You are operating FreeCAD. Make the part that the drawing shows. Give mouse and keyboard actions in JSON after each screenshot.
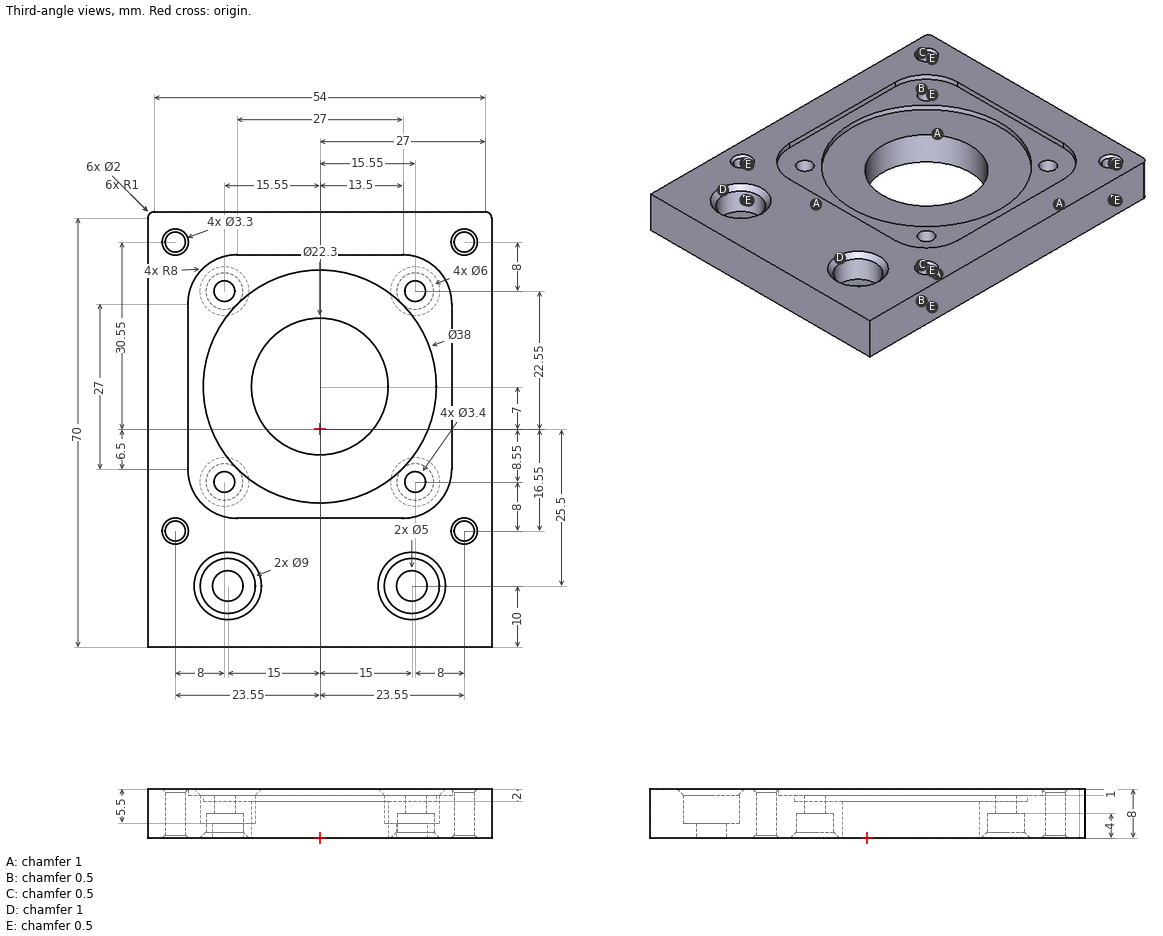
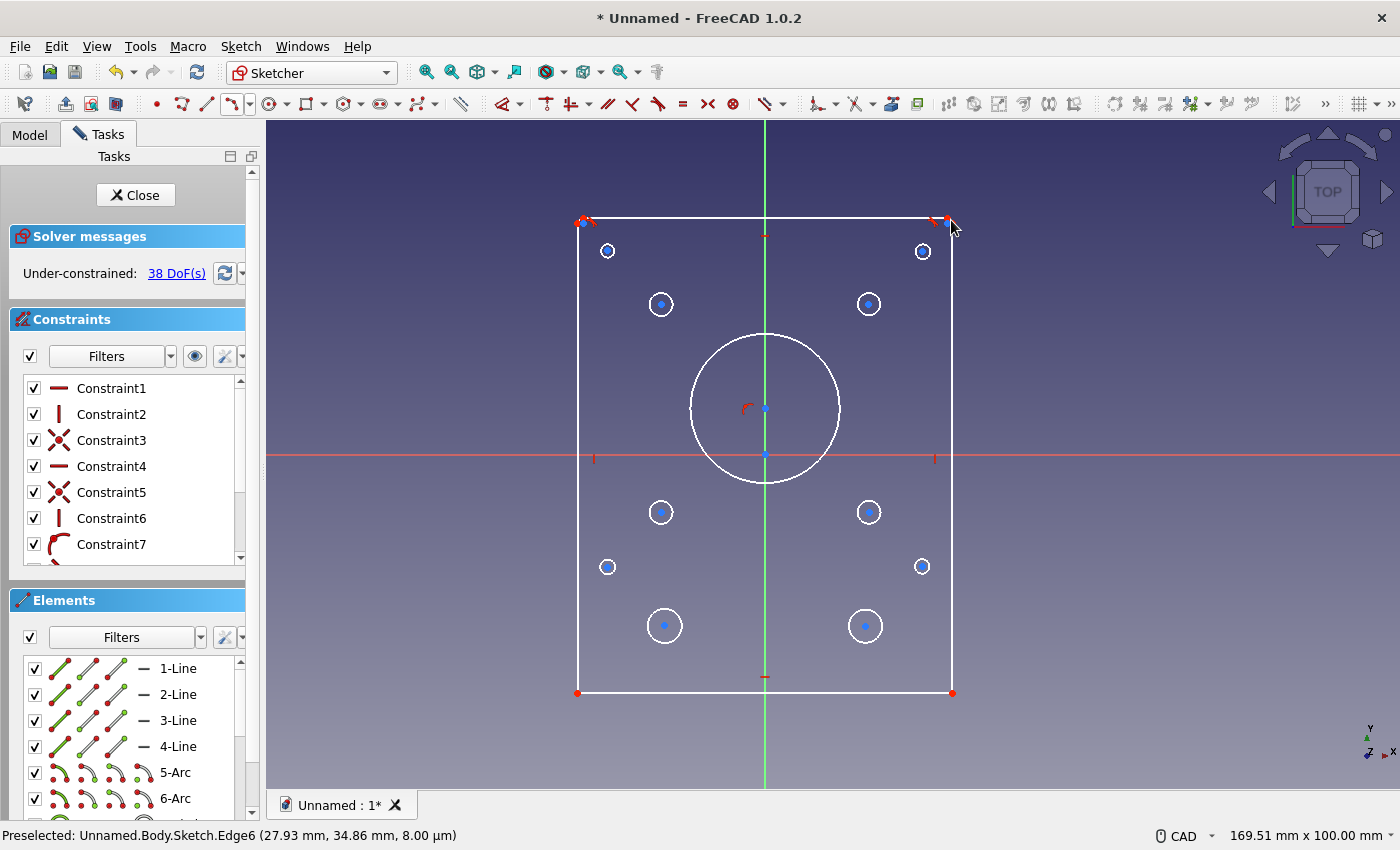
{"action": "scroll", "coordinate": [579, 220], "scroll_direction": "up", "scroll_amount": 7}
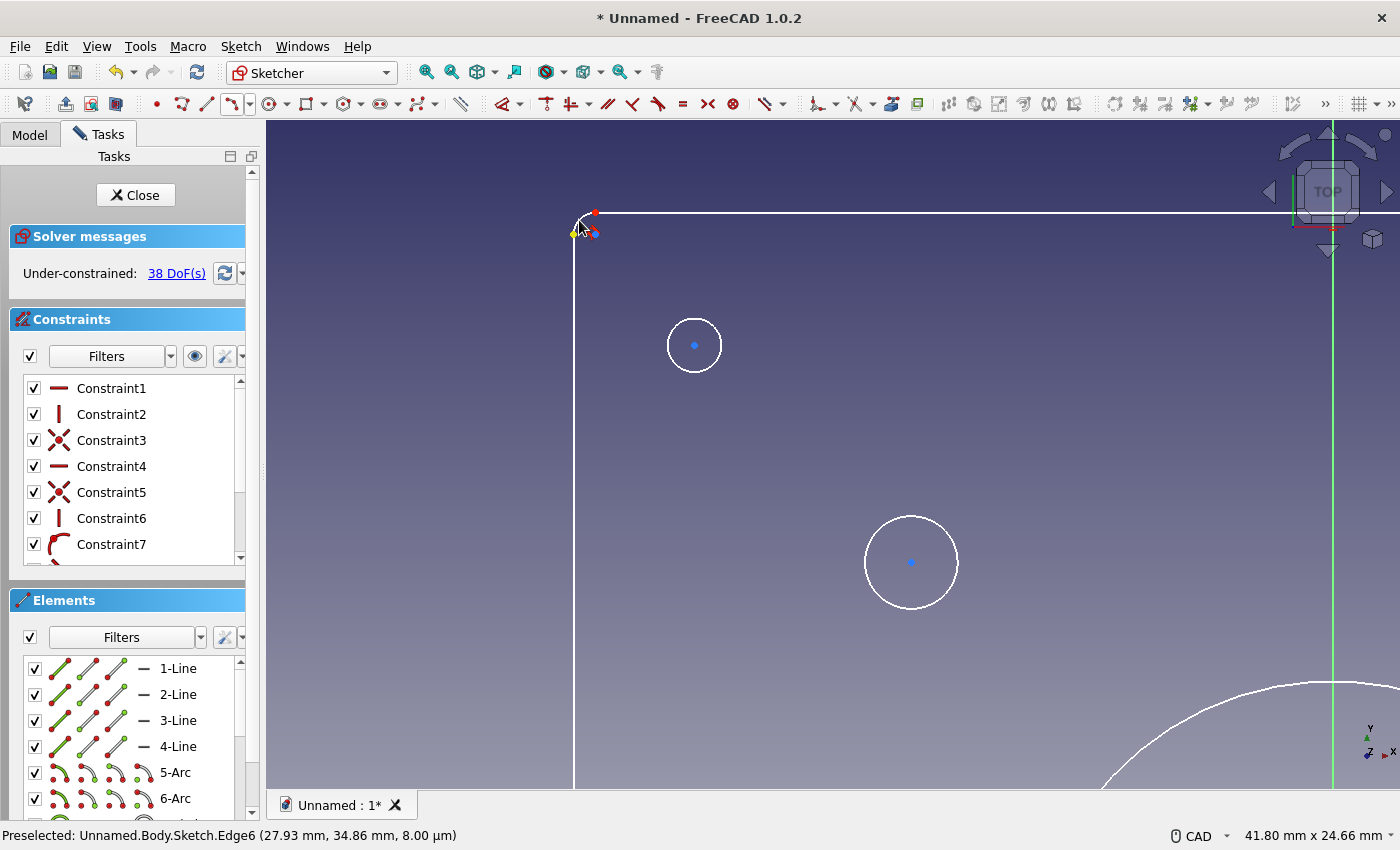
{"action": "left_click", "coordinate": [580, 219]}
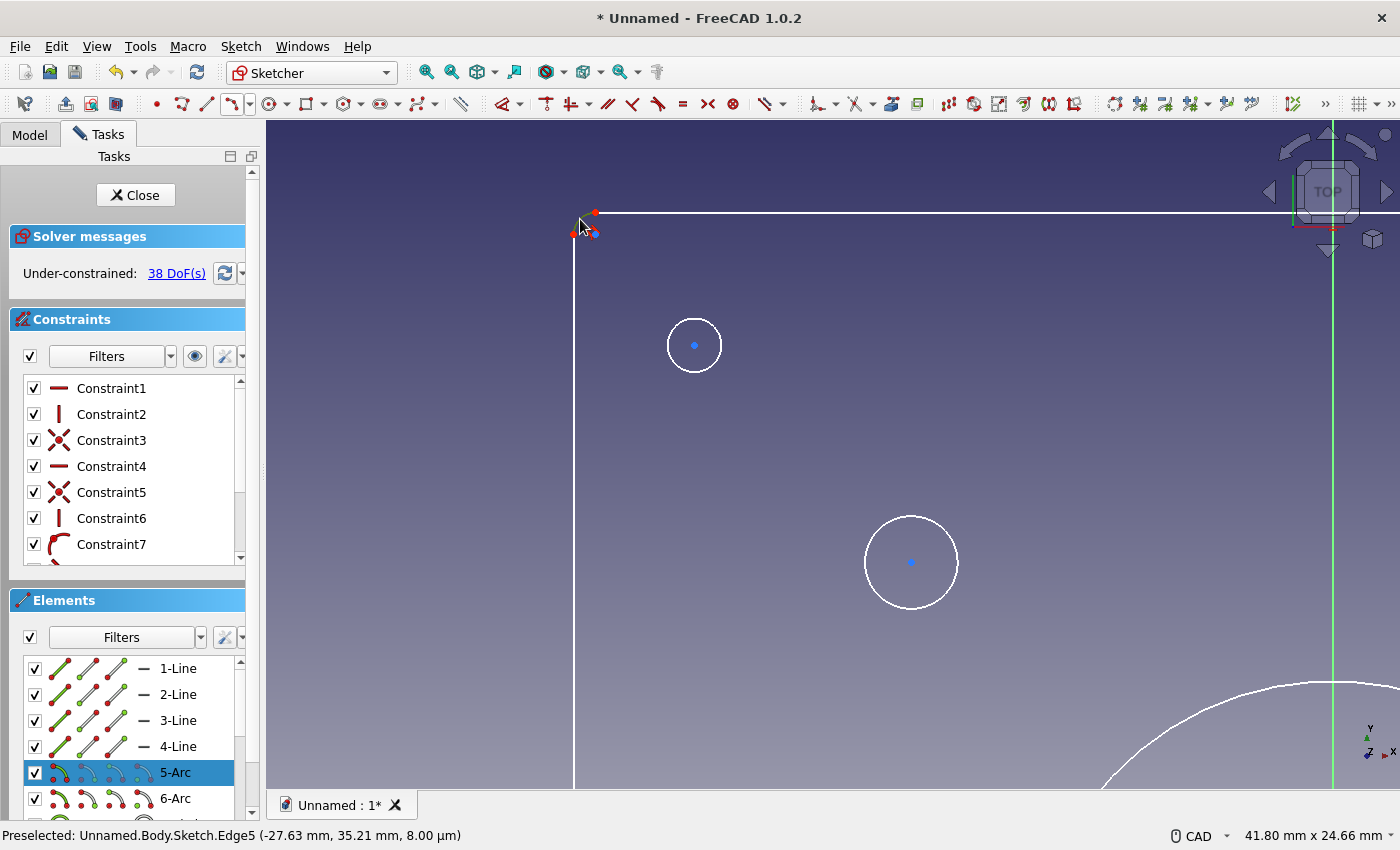
{"action": "scroll", "coordinate": [578, 220], "scroll_direction": "down", "scroll_amount": 7}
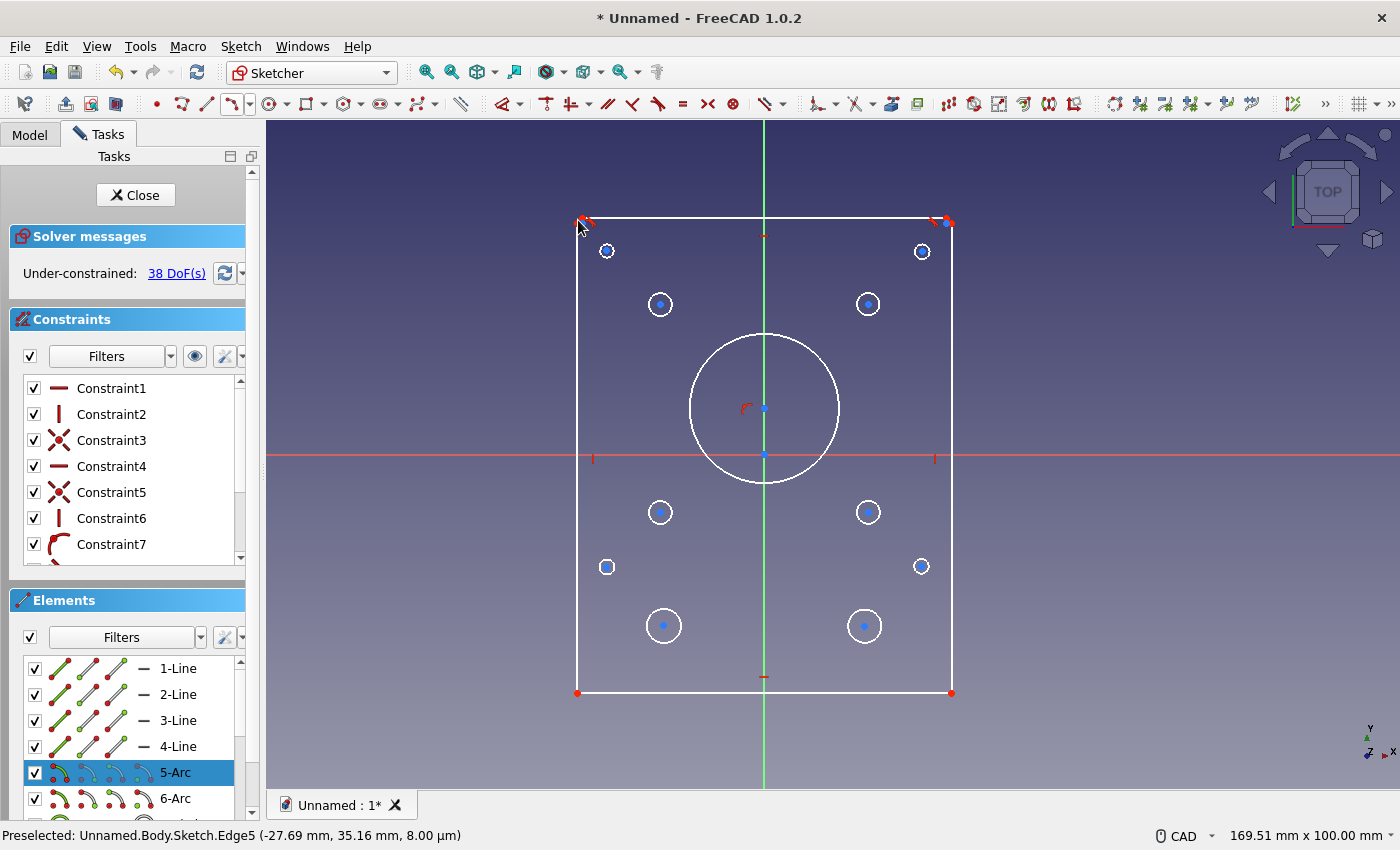
{"action": "scroll", "coordinate": [951, 221], "scroll_direction": "up", "scroll_amount": 9}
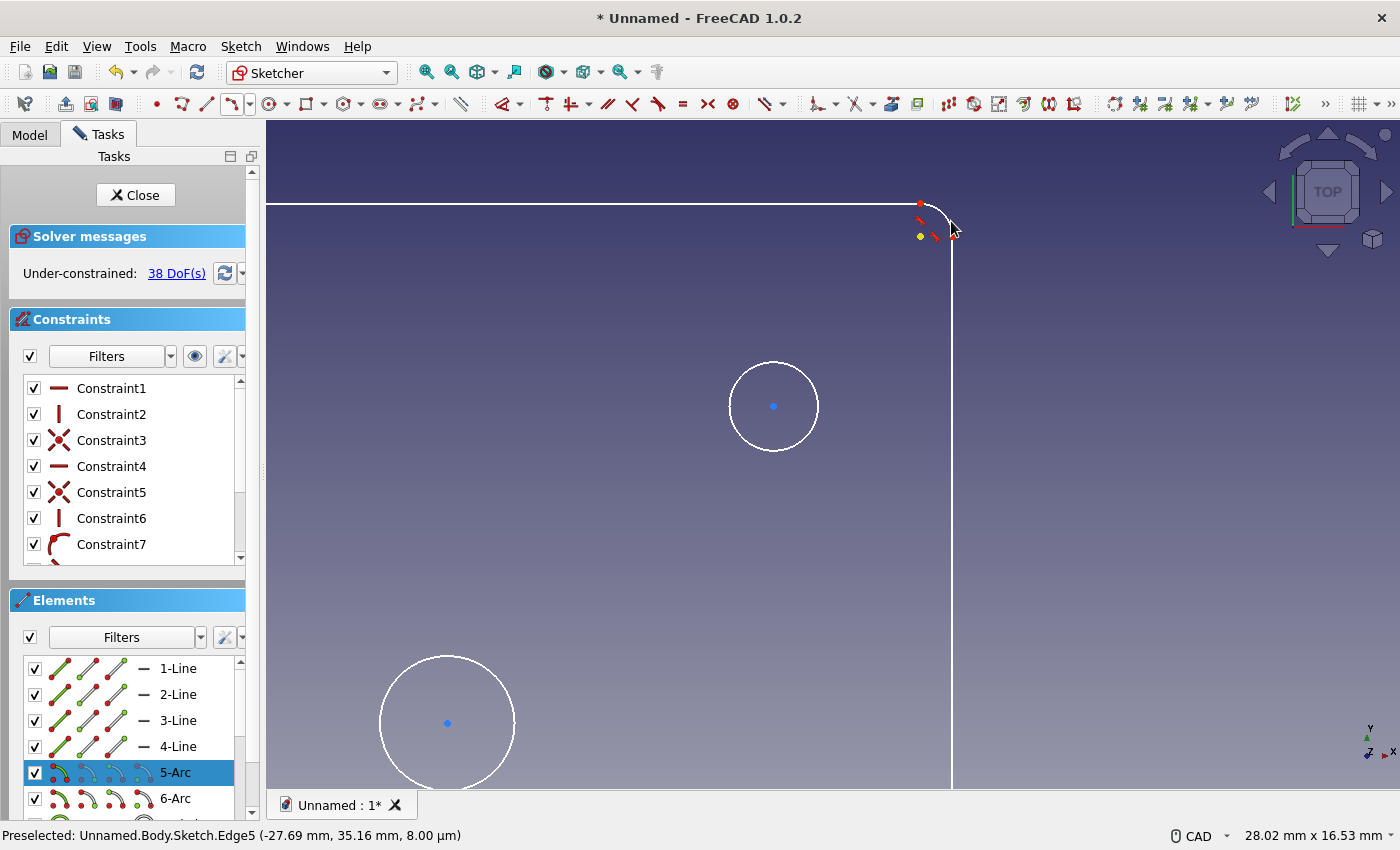
{"action": "left_click", "coordinate": [949, 222]}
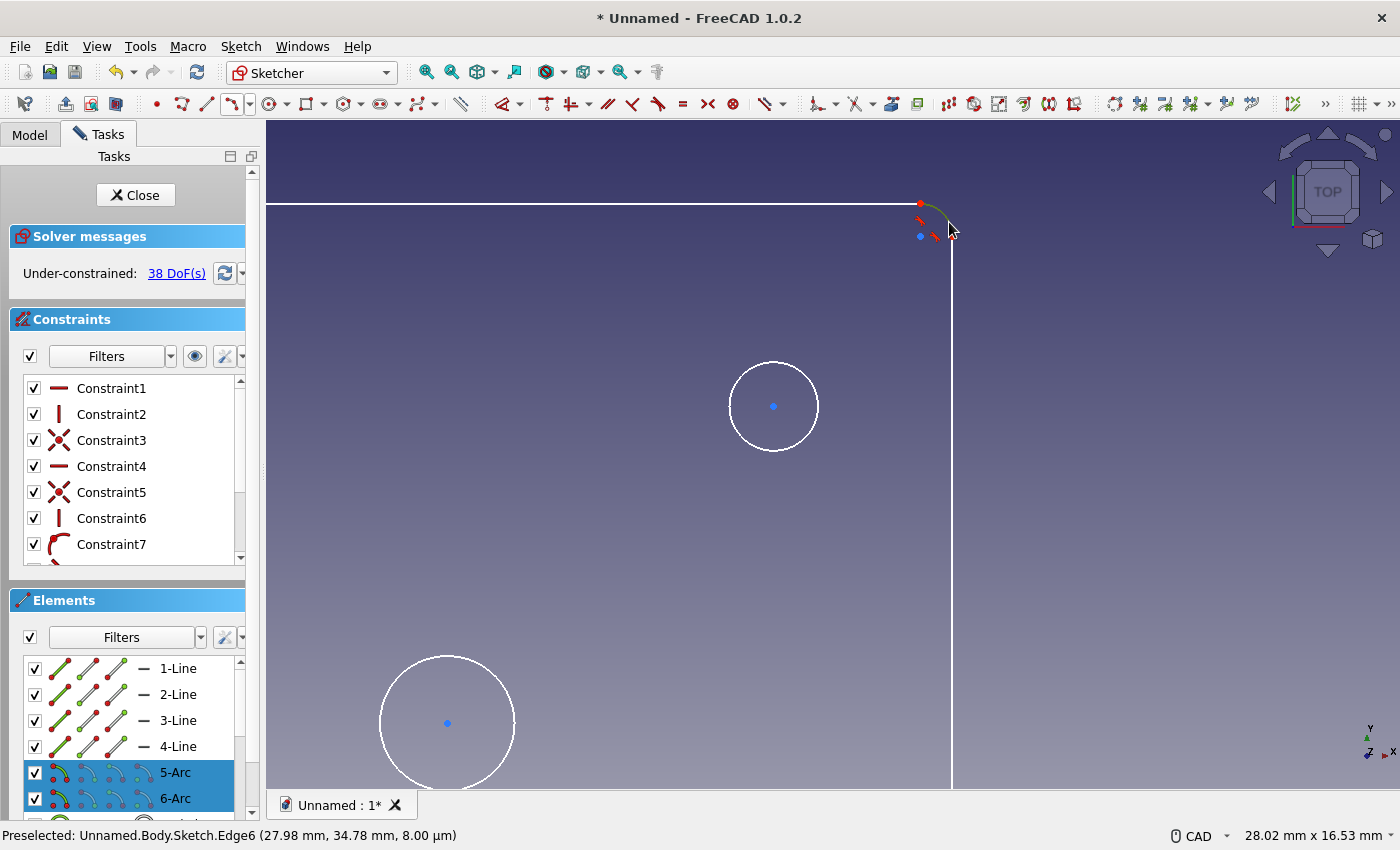
{"action": "left_click", "coordinate": [683, 104]}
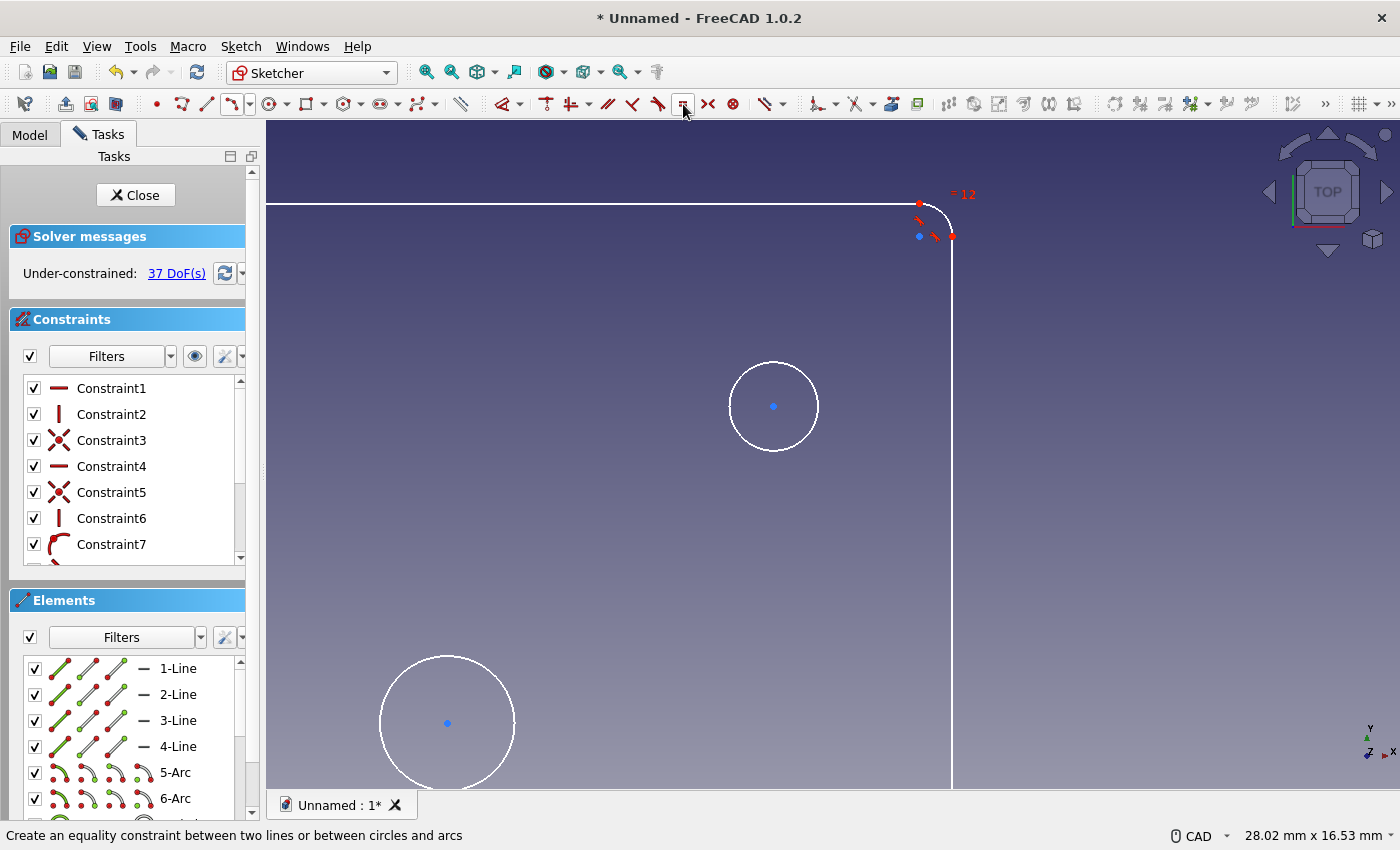
{"action": "scroll", "coordinate": [952, 221], "scroll_direction": "down", "scroll_amount": 9}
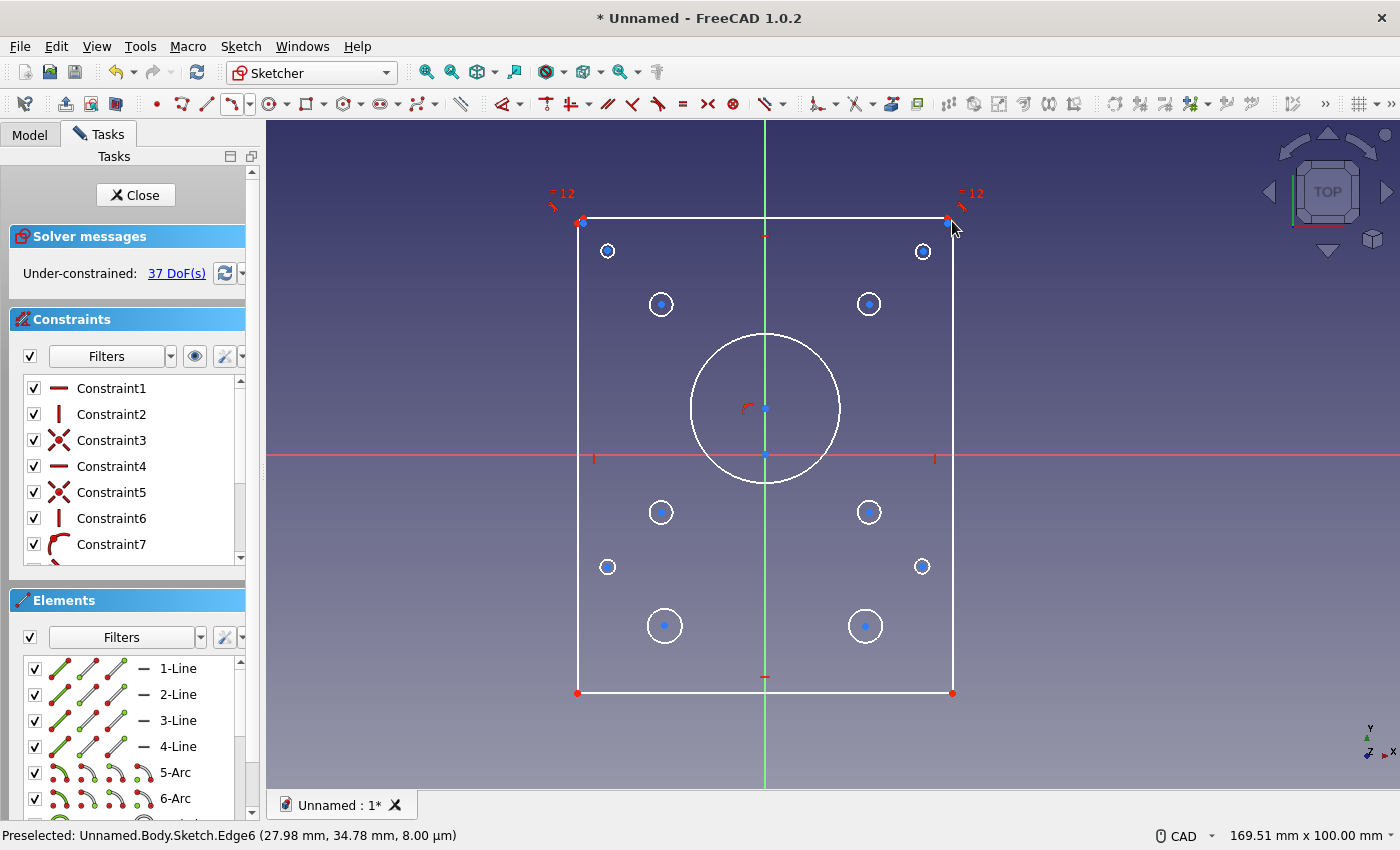
{"action": "left_click", "coordinate": [877, 614]}